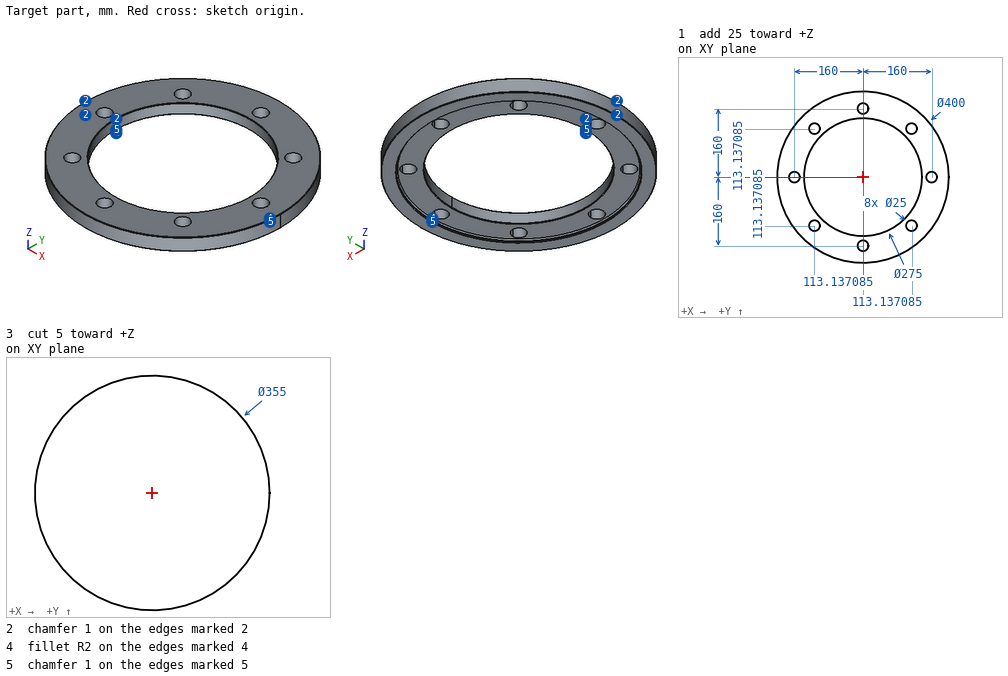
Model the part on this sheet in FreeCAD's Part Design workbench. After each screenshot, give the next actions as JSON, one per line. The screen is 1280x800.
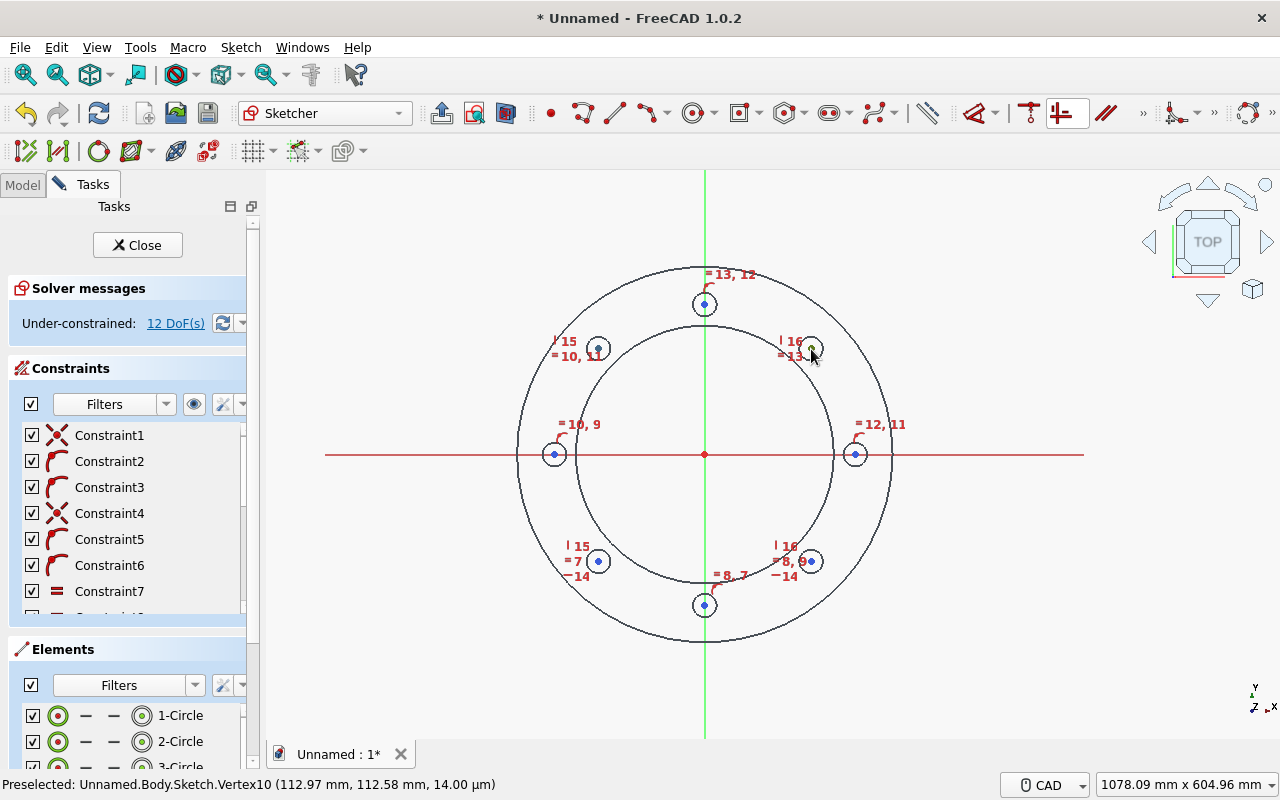
{"action": "left_click", "coordinate": [1084, 114]}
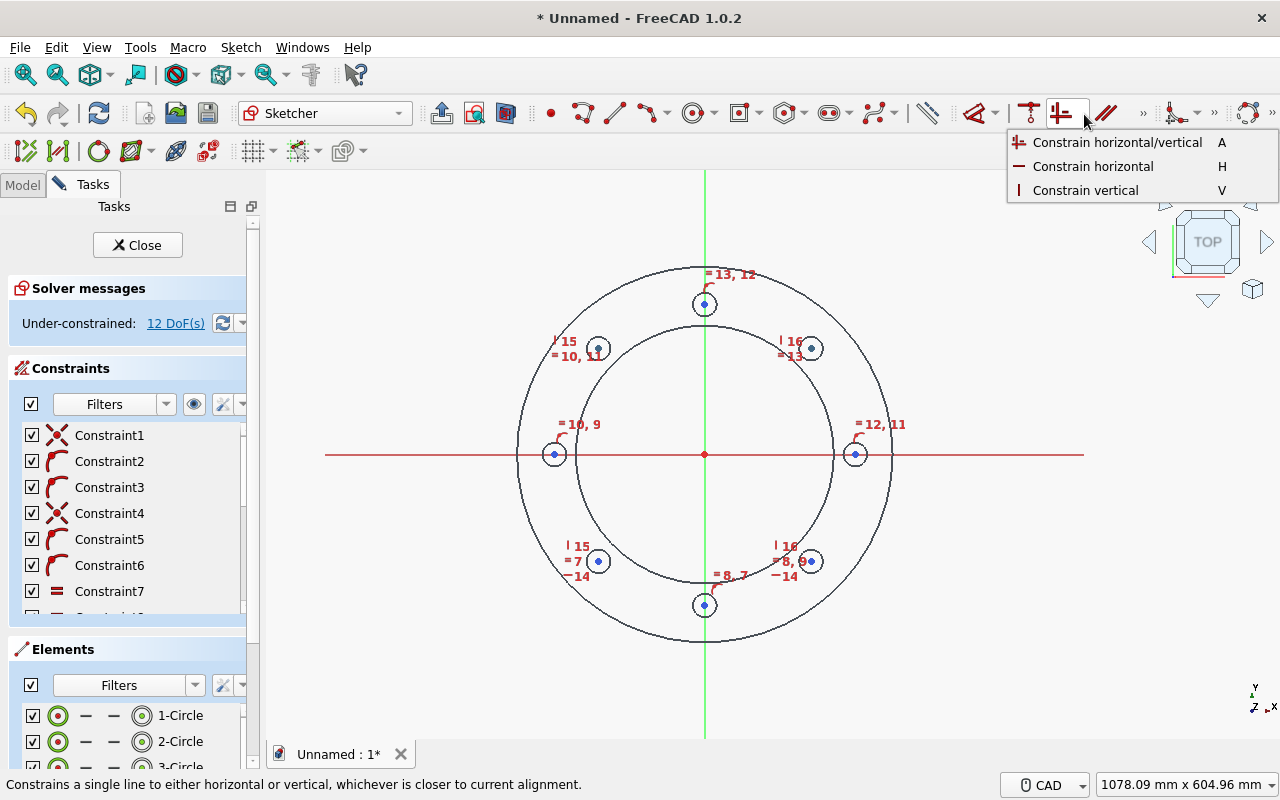
{"action": "left_click", "coordinate": [1143, 166]}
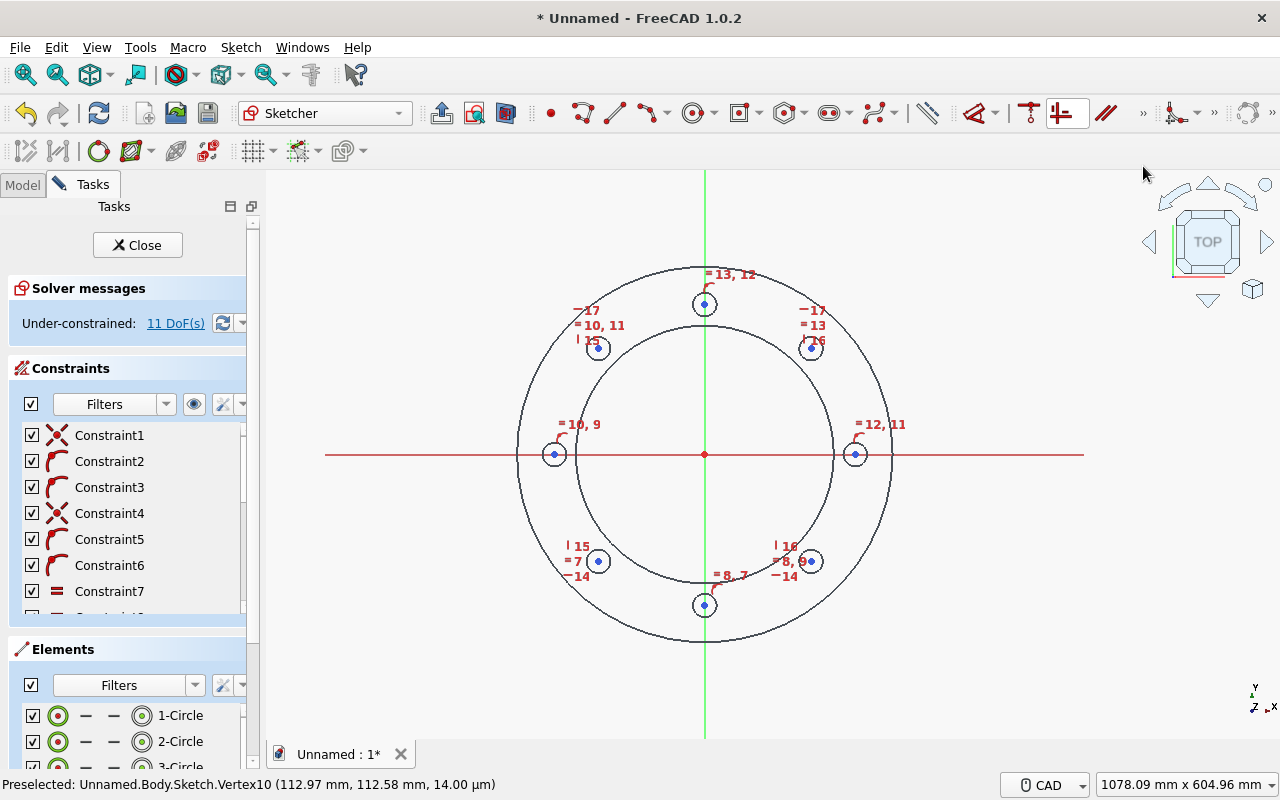
{"action": "left_click", "coordinate": [974, 114]}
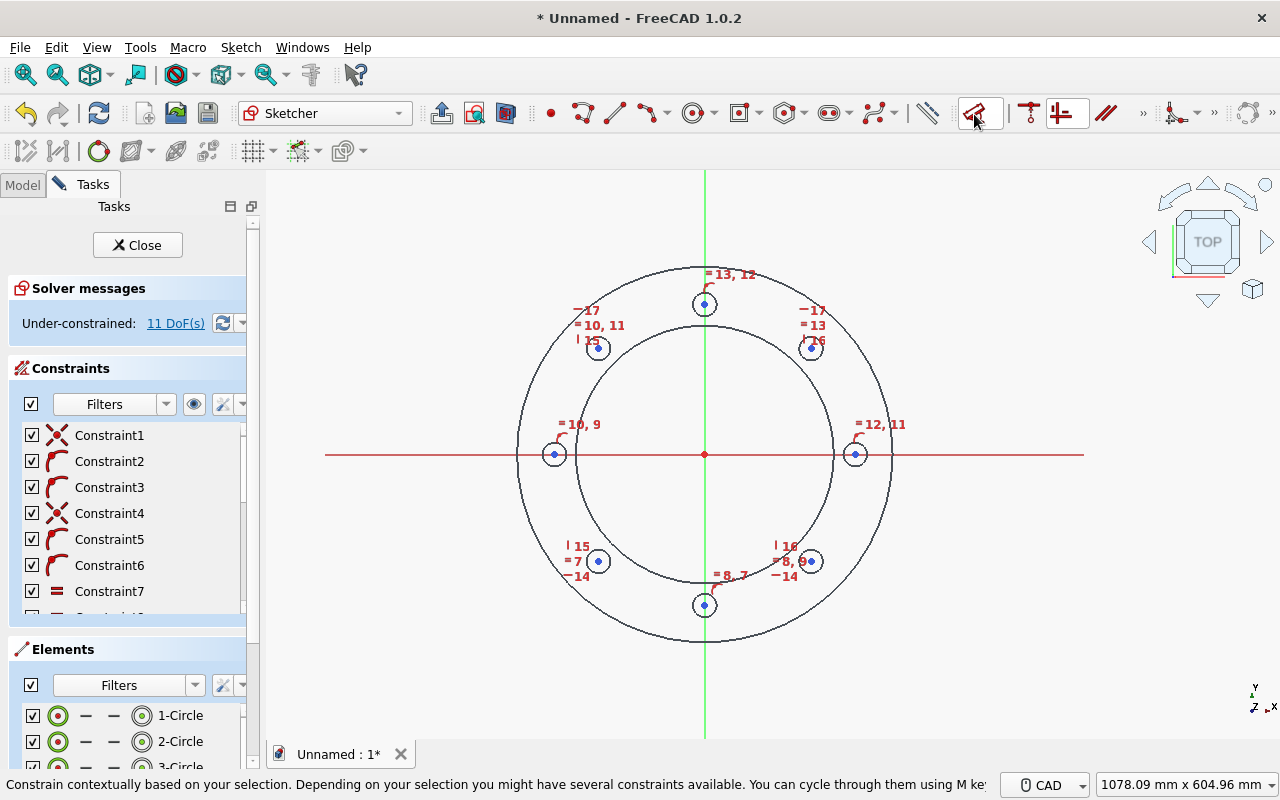
{"action": "left_click", "coordinate": [837, 321]}
{"action": "left_click", "coordinate": [860, 298]}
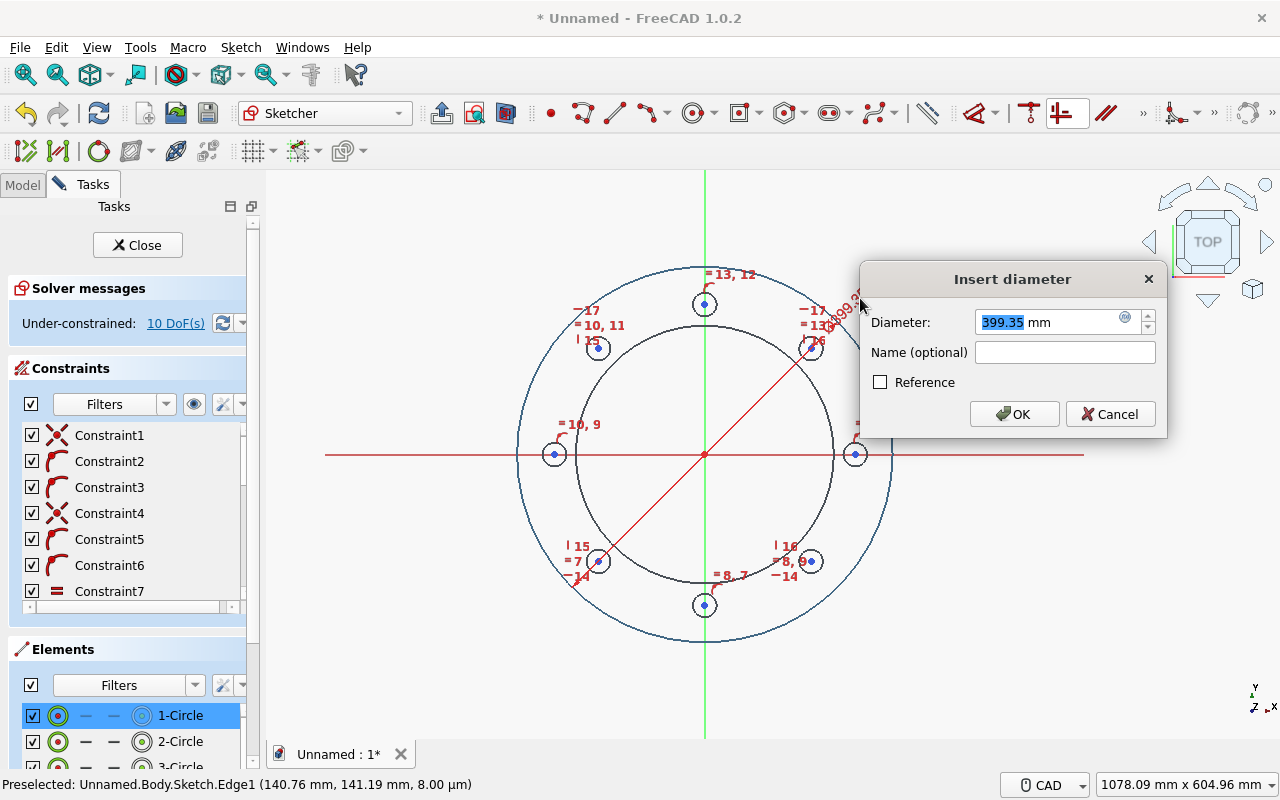
{"action": "type", "text": "400"}
{"action": "key", "text": "Return"}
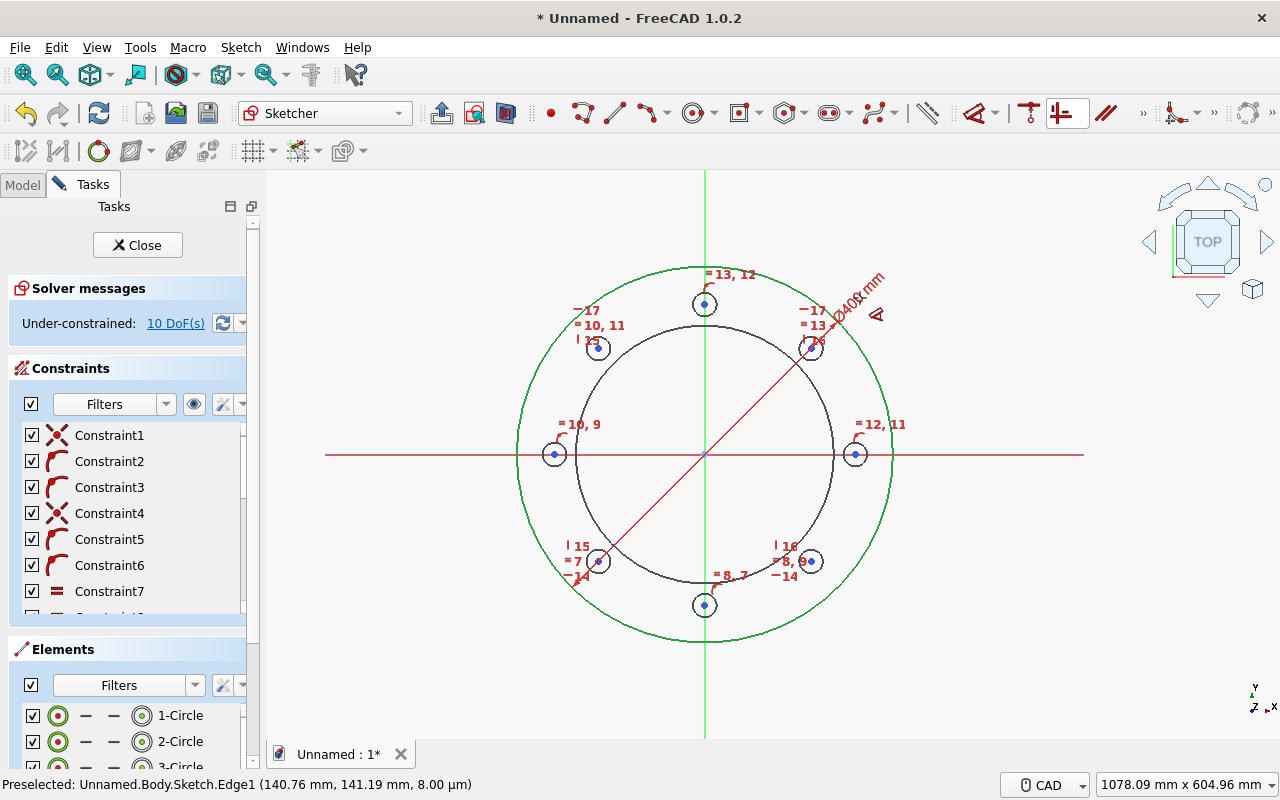
{"action": "scroll", "coordinate": [607, 553], "scroll_direction": "up", "scroll_amount": 3}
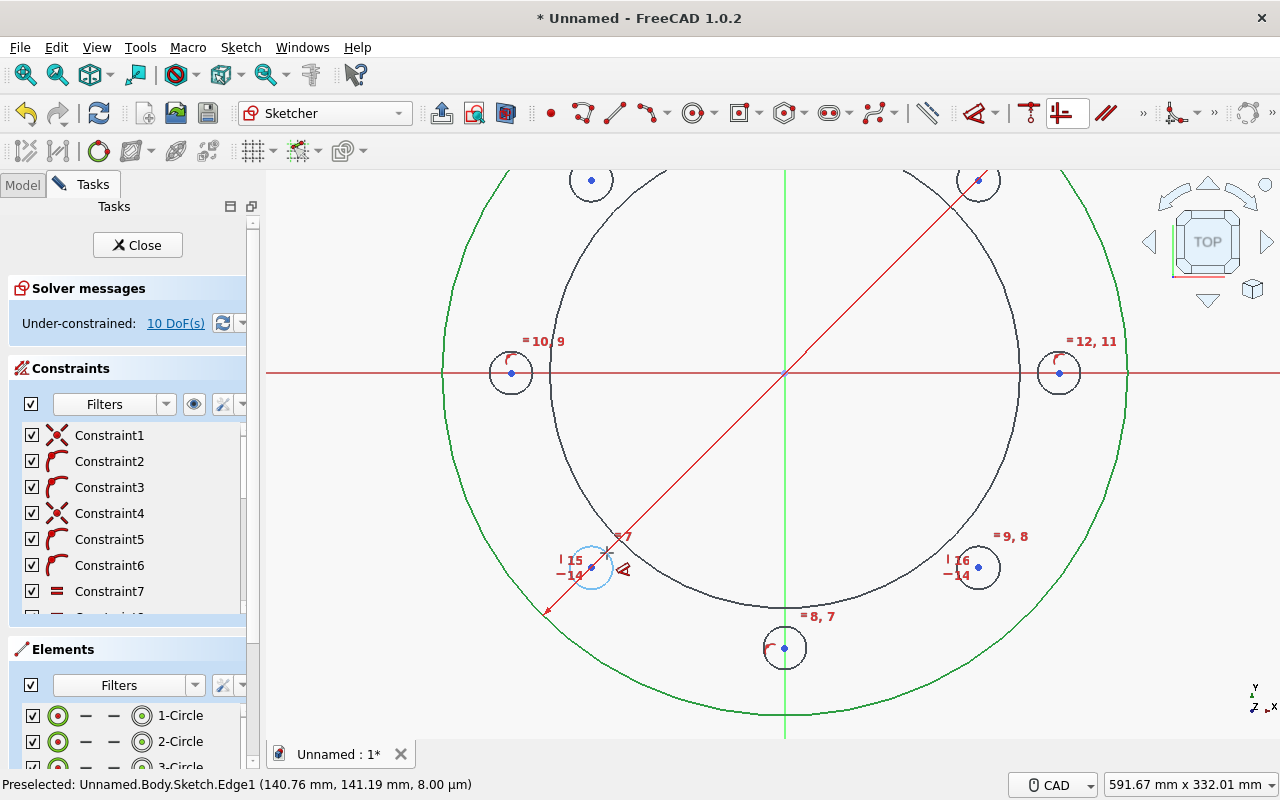
{"action": "left_click", "coordinate": [606, 553]}
{"action": "left_click", "coordinate": [629, 530]}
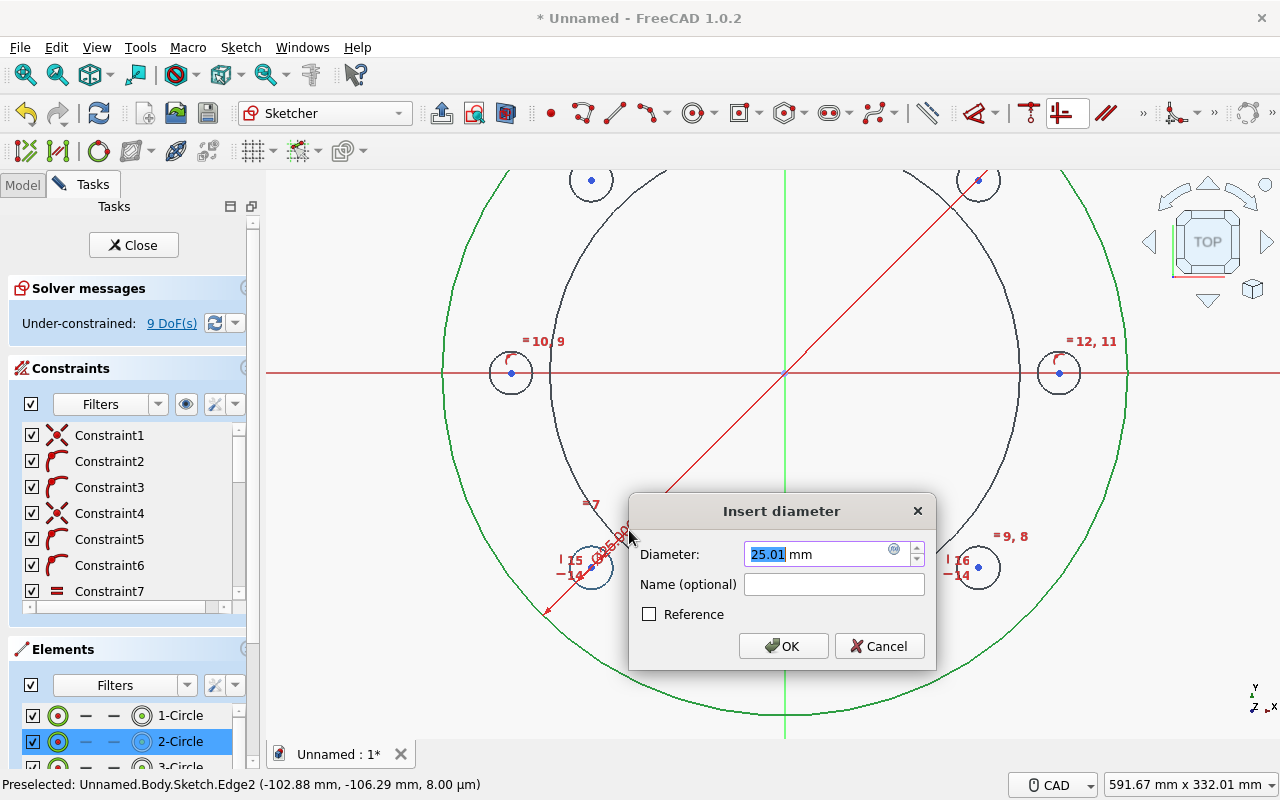
{"action": "type", "text": "25"}
{"action": "key", "text": "Return"}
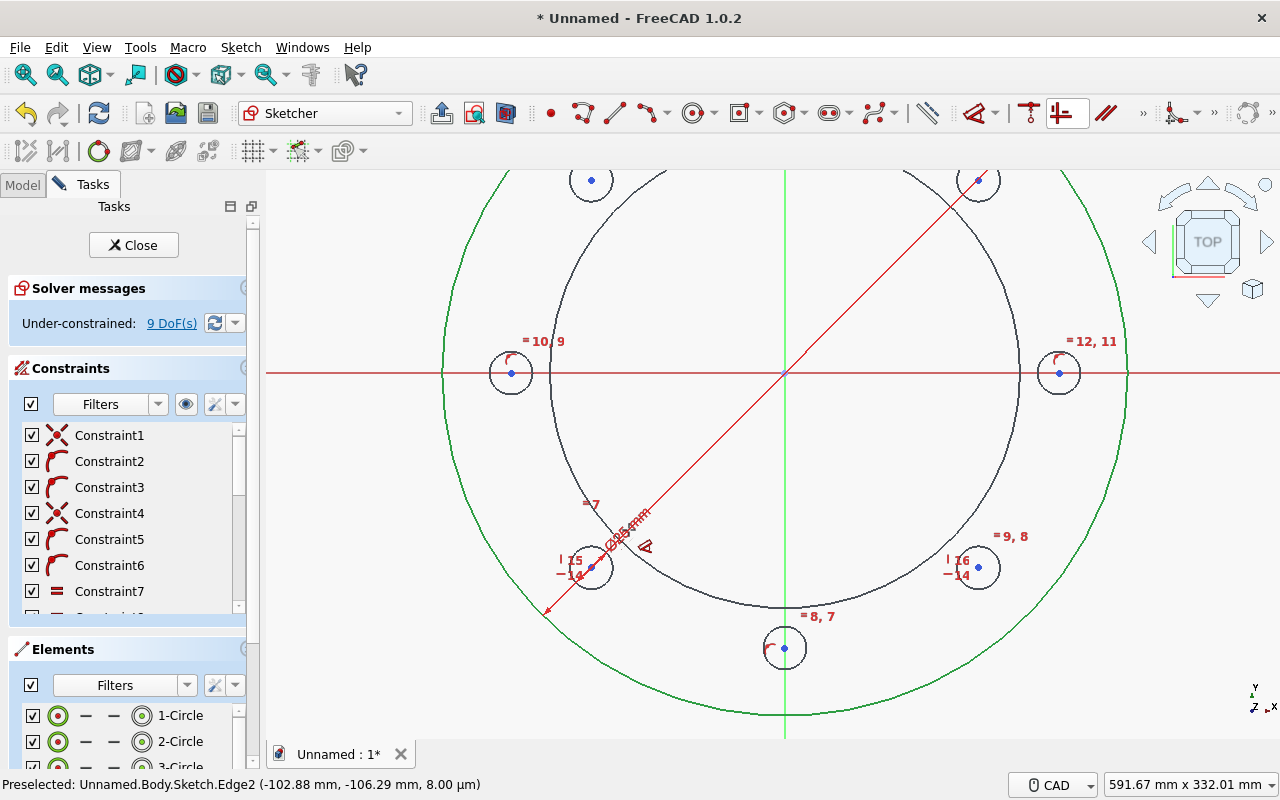
{"action": "left_click", "coordinate": [951, 206]}
{"action": "left_click", "coordinate": [1041, 297]}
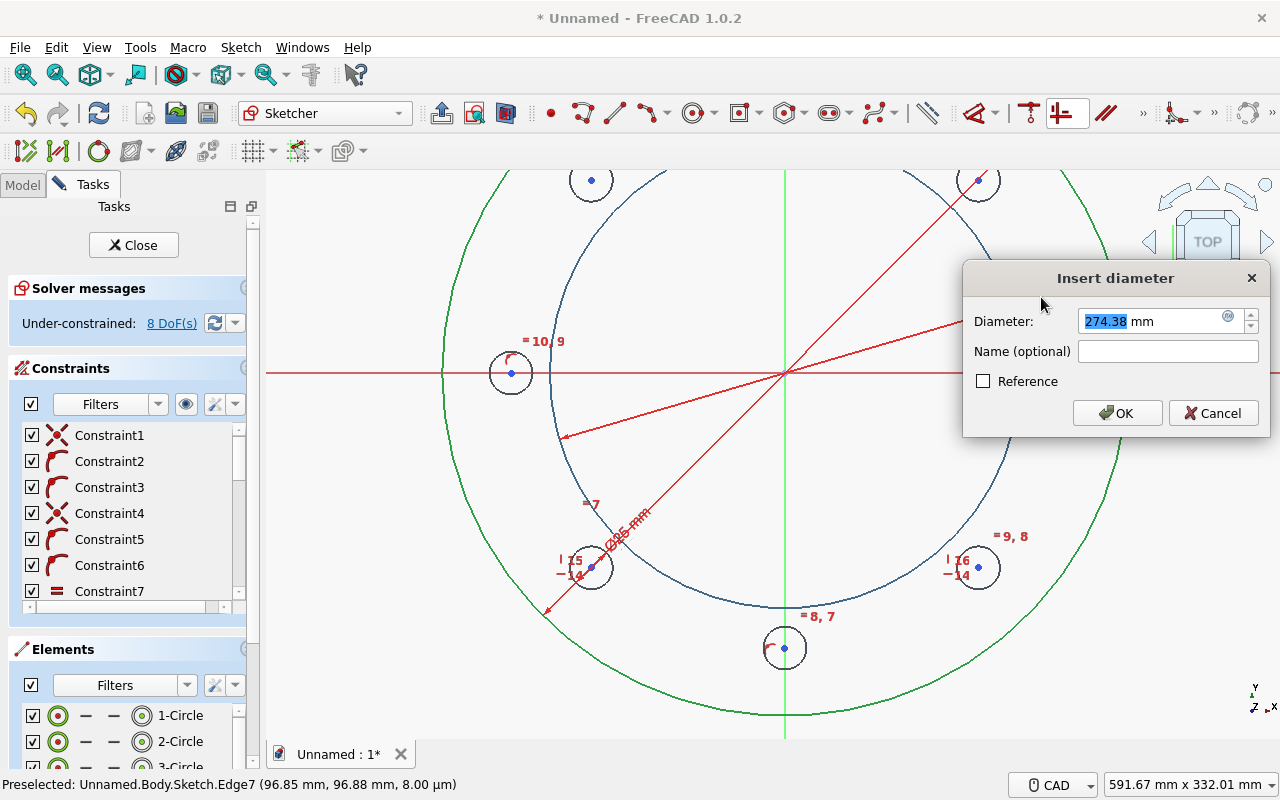
{"action": "type", "text": "275"}
{"action": "key", "text": "Return"}